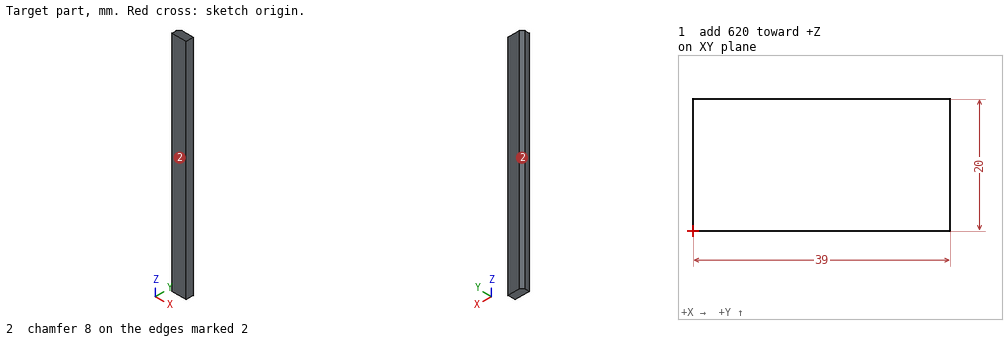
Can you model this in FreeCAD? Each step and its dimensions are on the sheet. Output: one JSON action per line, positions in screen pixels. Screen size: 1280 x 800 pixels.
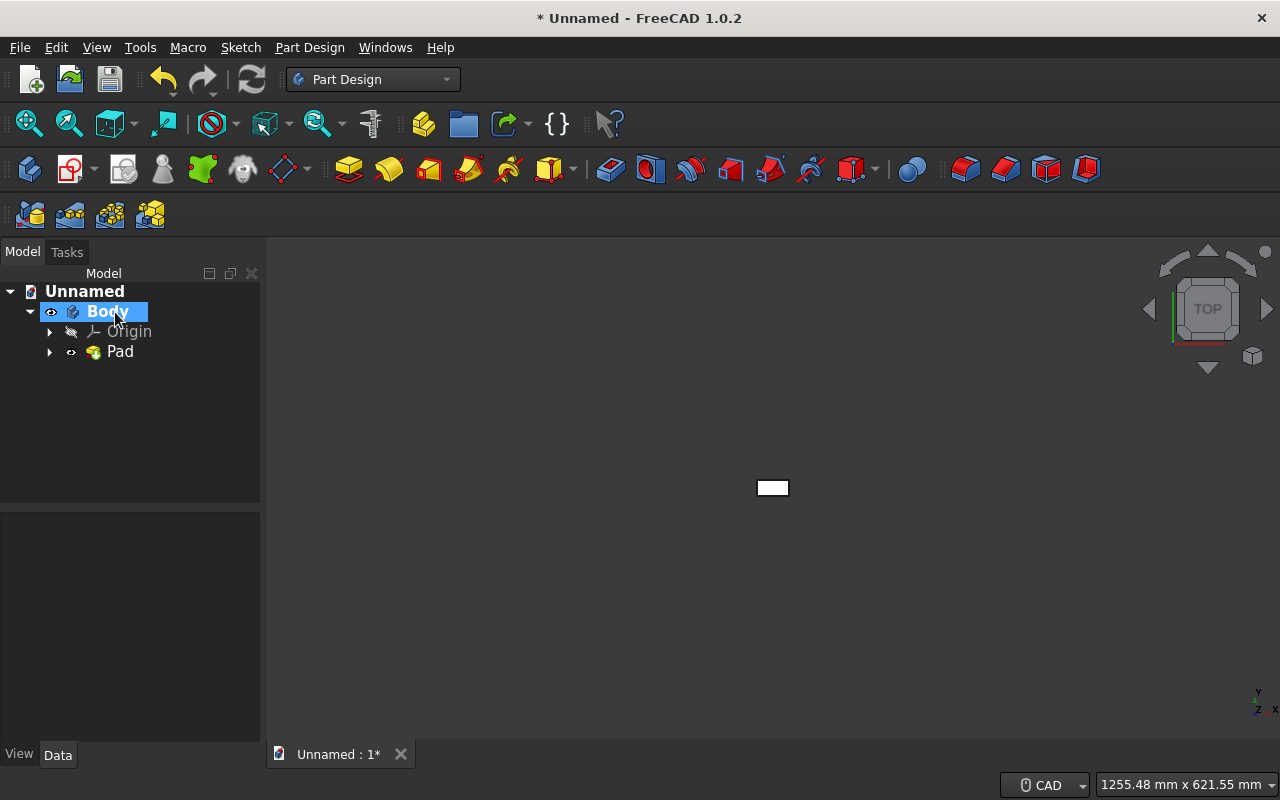
{"action": "key", "text": "1"}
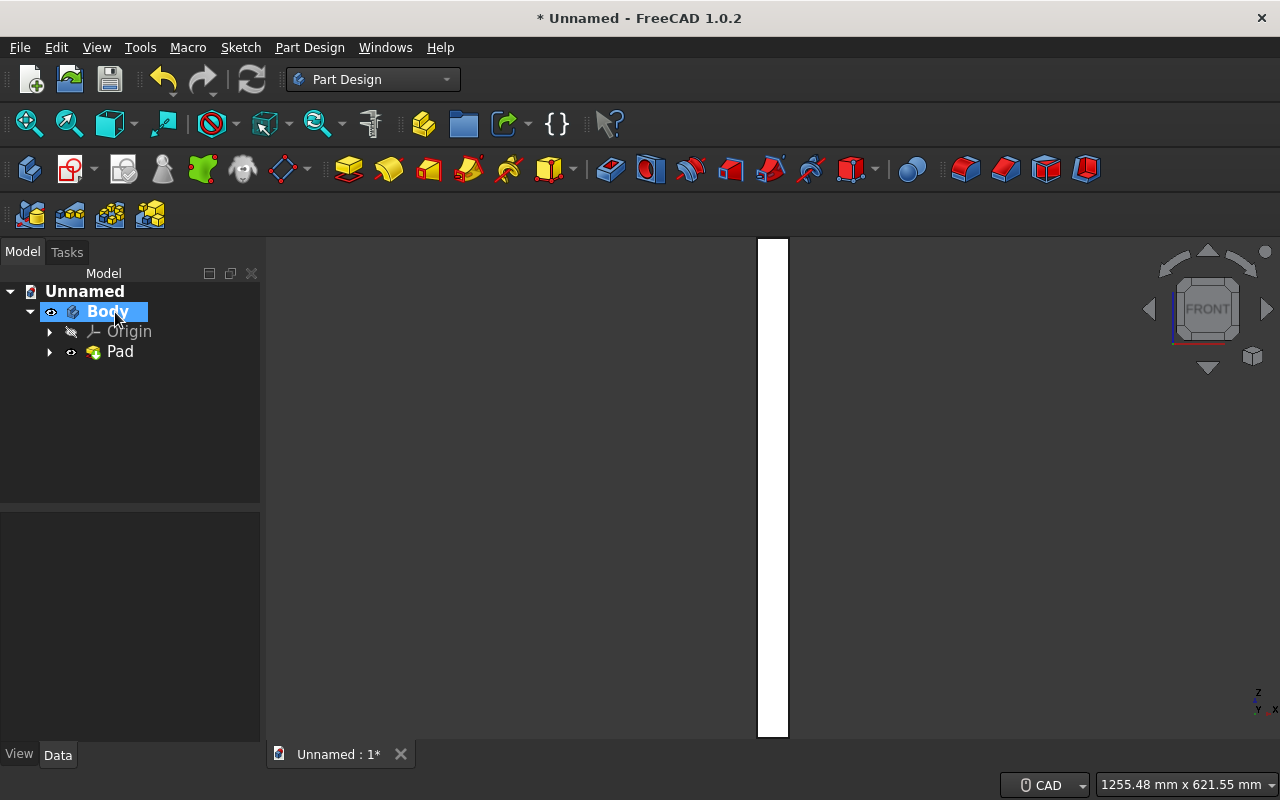
{"action": "key", "text": "3"}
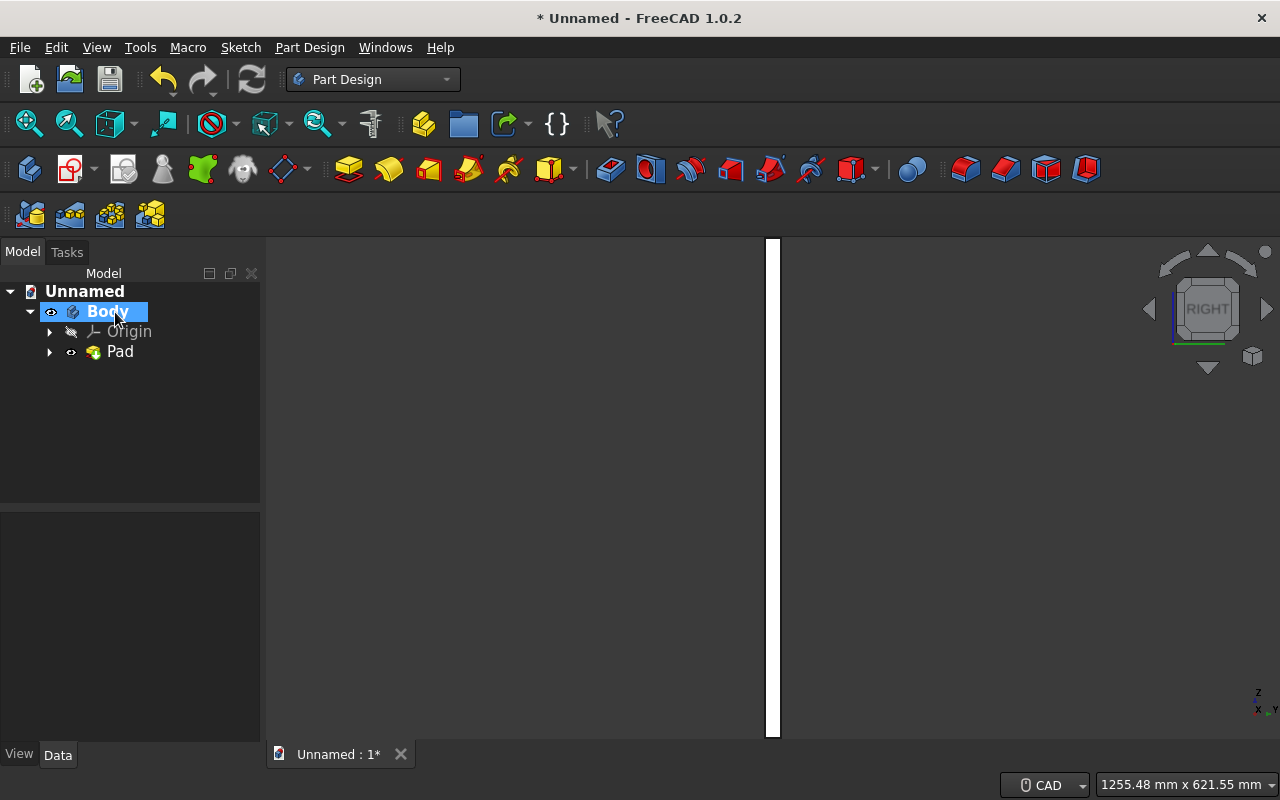
{"action": "key", "text": "5"}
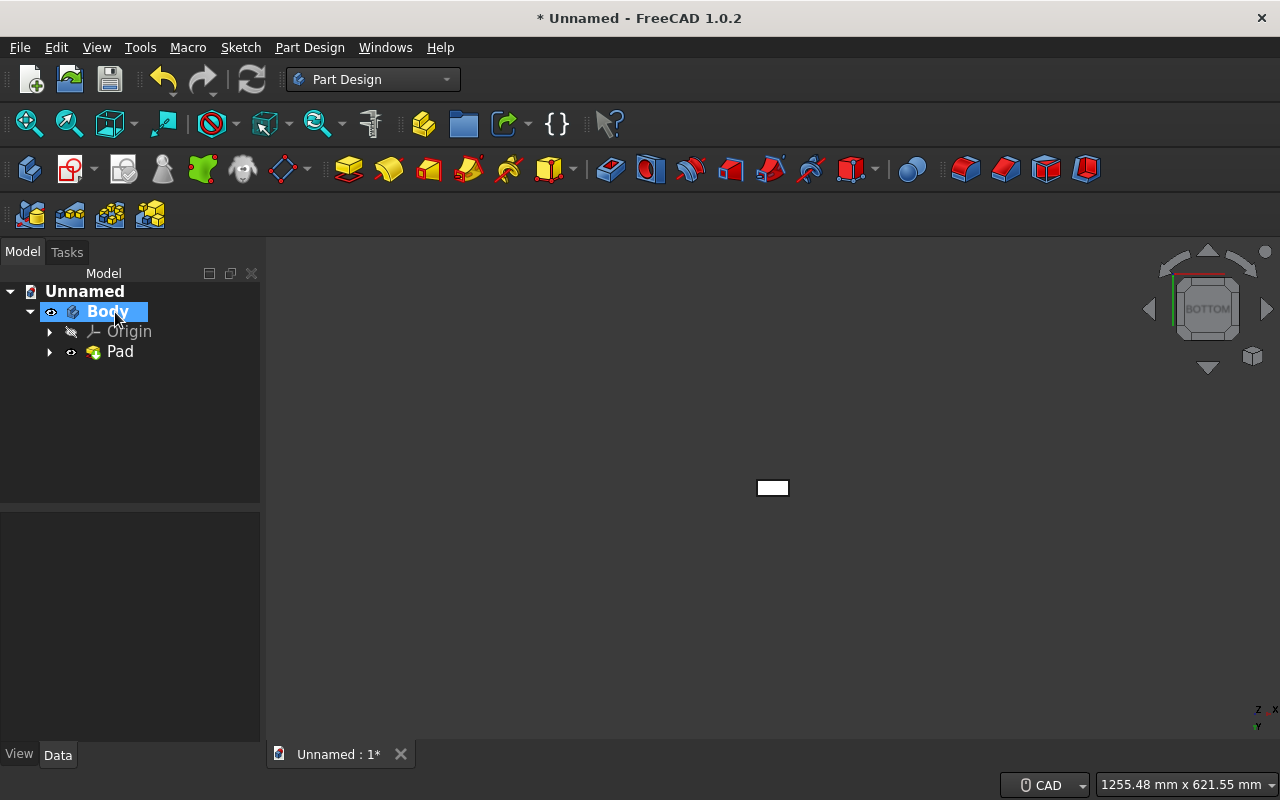
{"action": "left_click", "coordinate": [30, 124]}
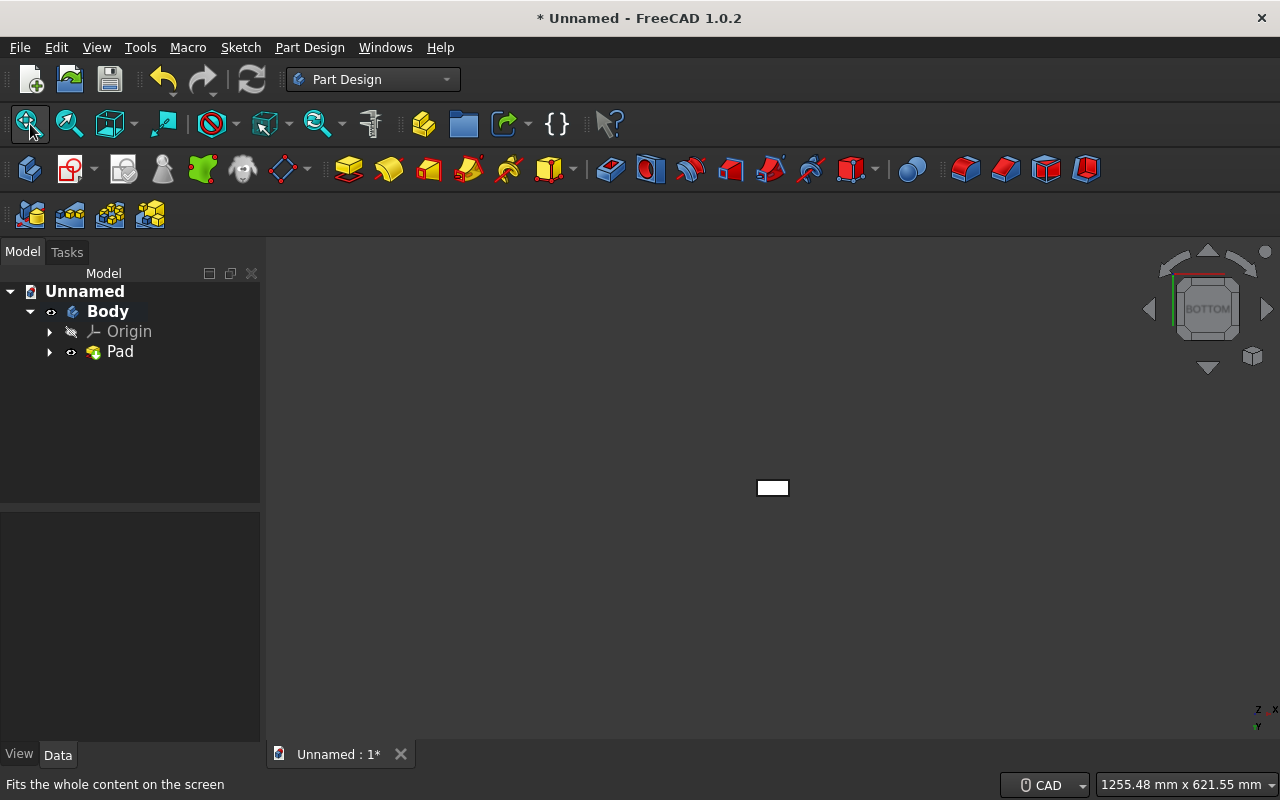
{"action": "key", "text": "4"}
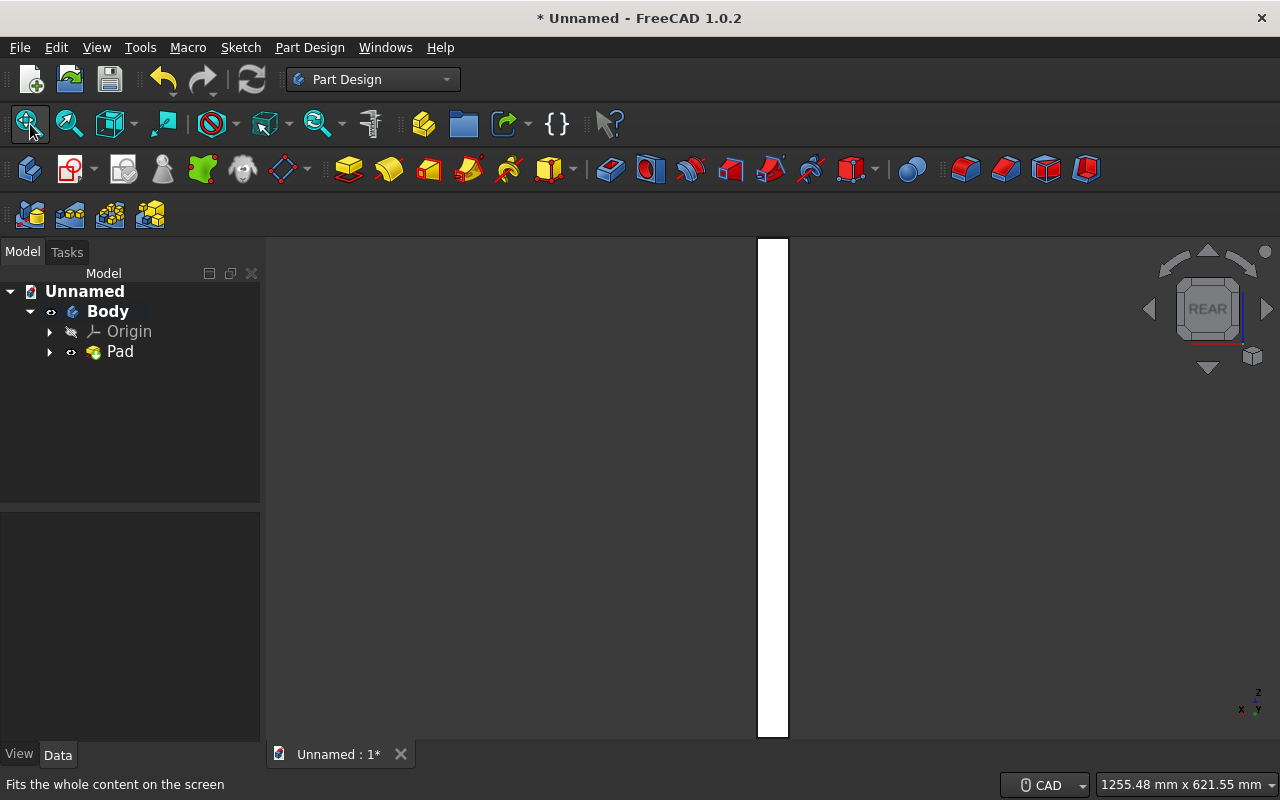
{"action": "left_click", "coordinate": [789, 487]}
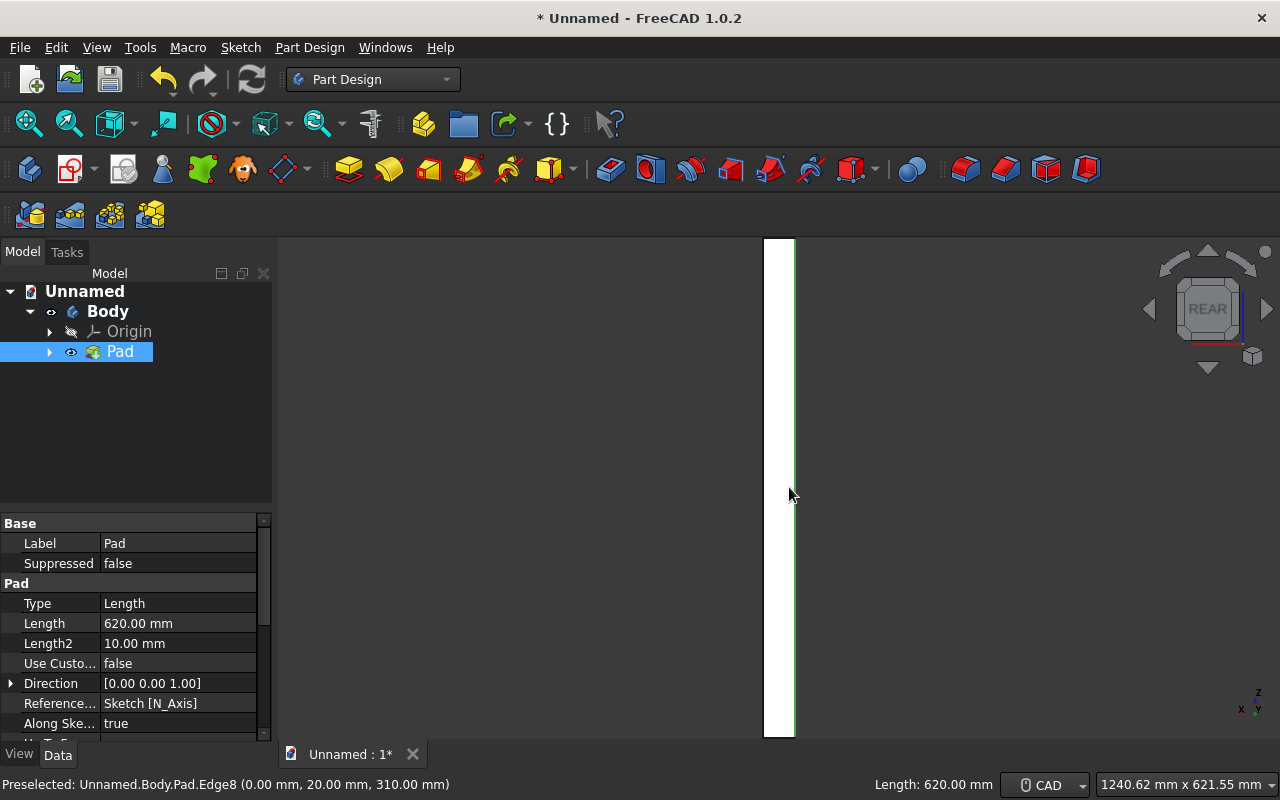
{"action": "left_click", "coordinate": [1006, 170]}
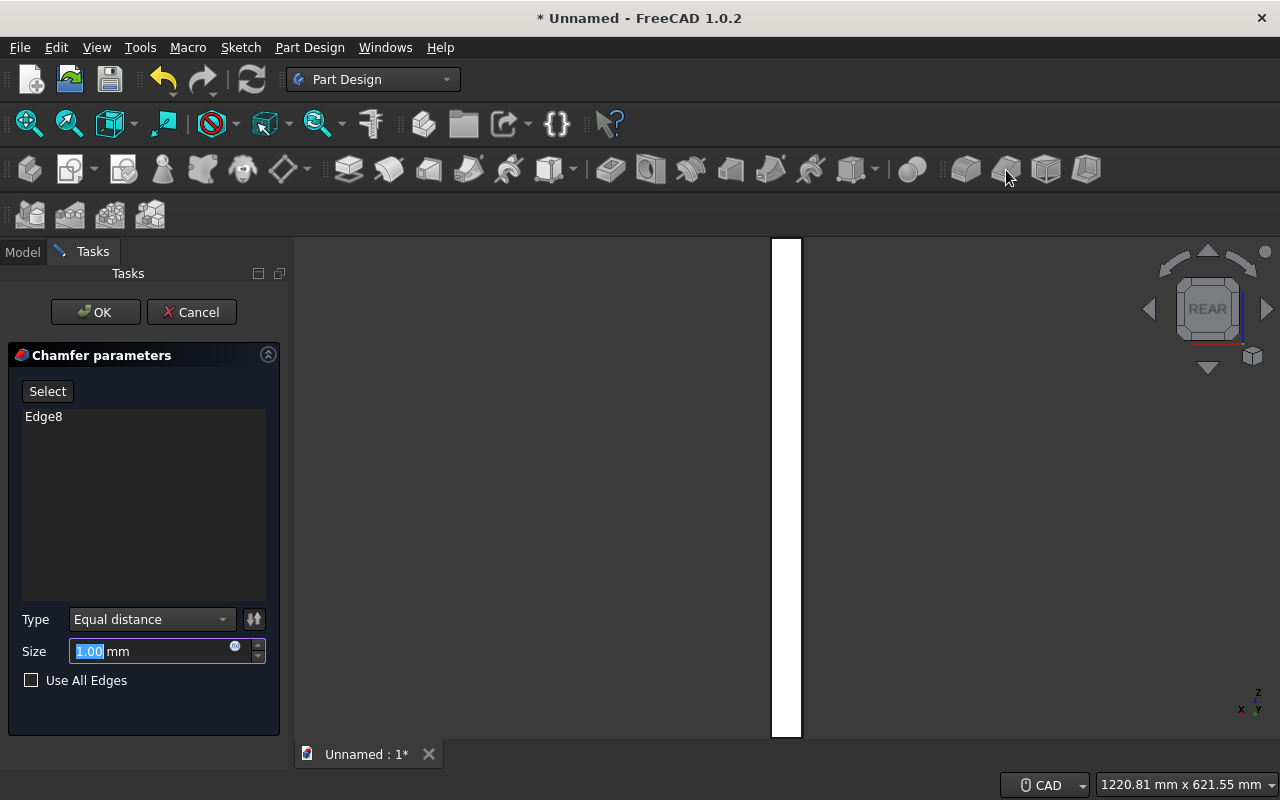
{"action": "type", "text": "8"}
{"action": "key", "text": "Tab"}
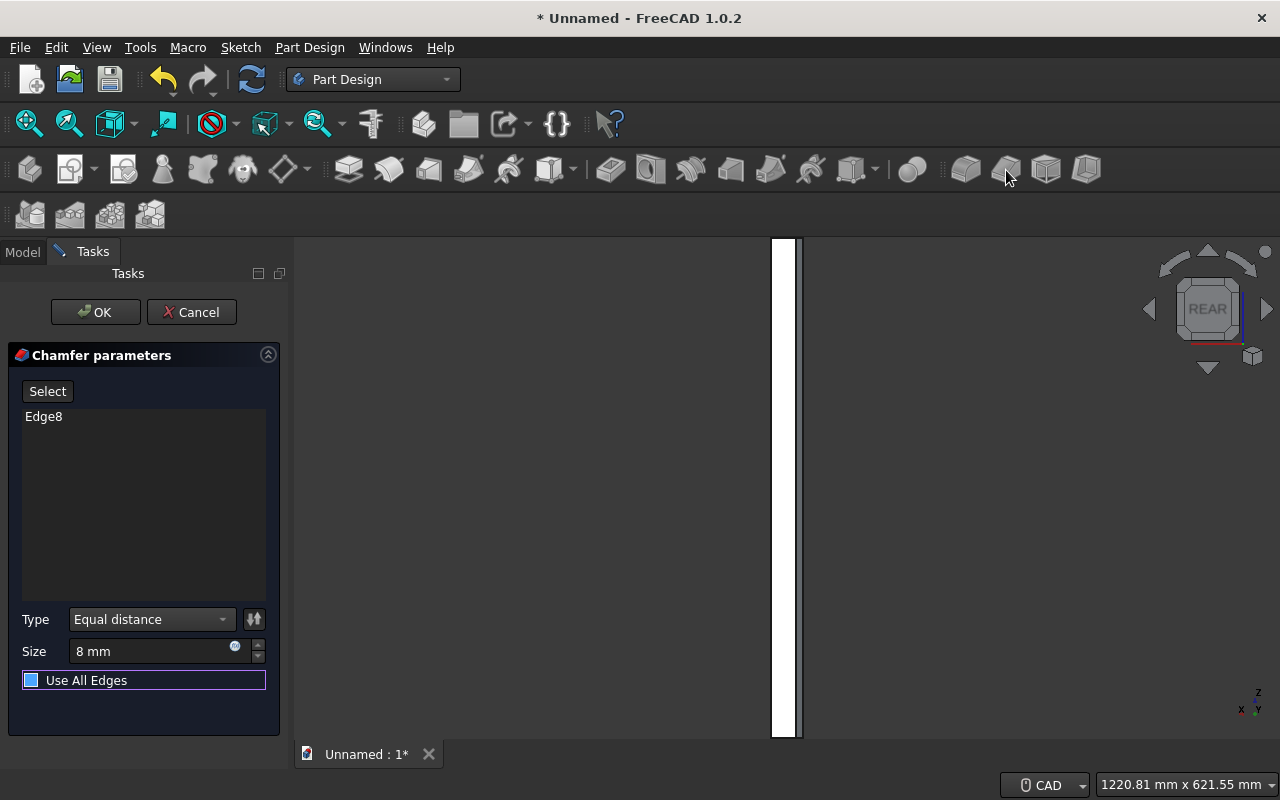
{"action": "left_click", "coordinate": [96, 312]}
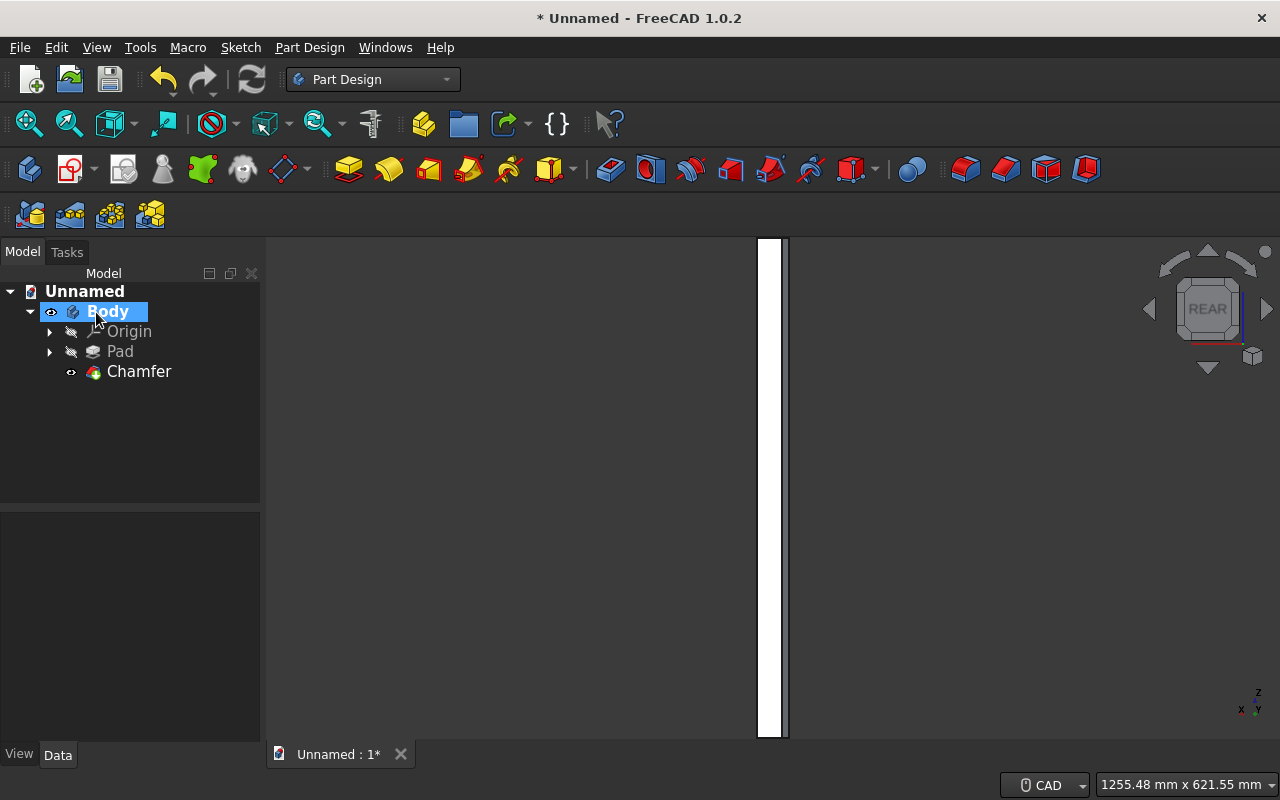
{"action": "key", "text": "0"}